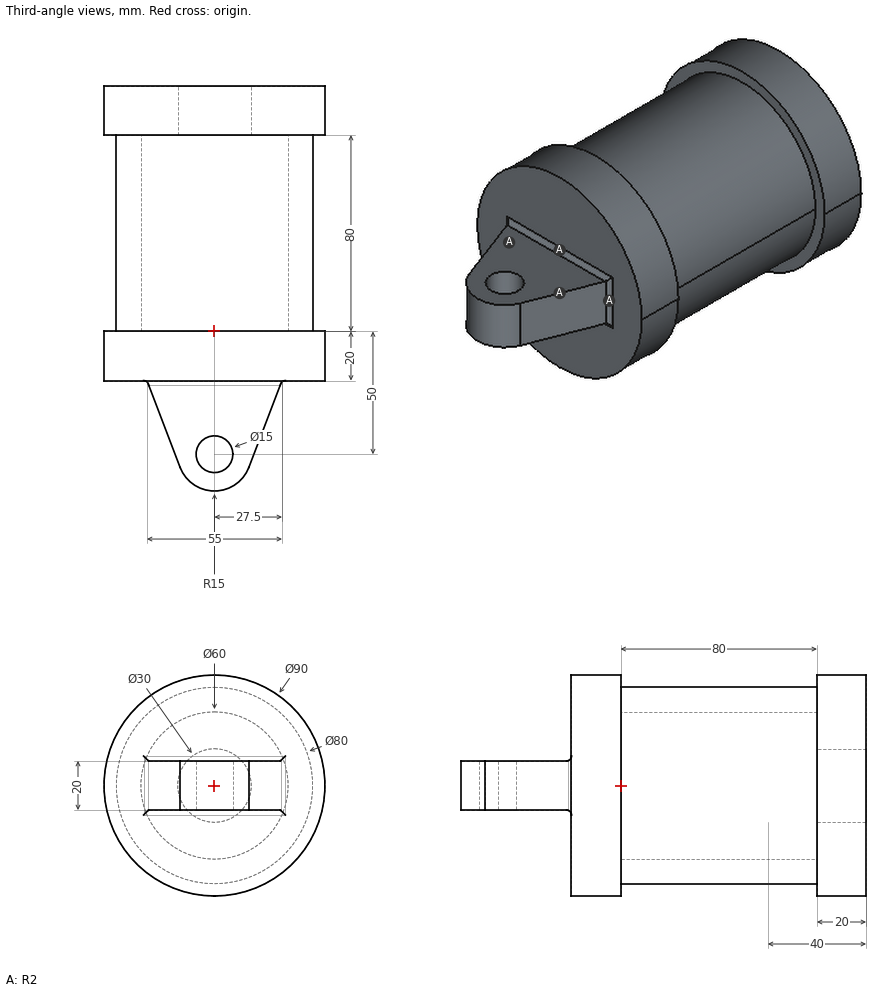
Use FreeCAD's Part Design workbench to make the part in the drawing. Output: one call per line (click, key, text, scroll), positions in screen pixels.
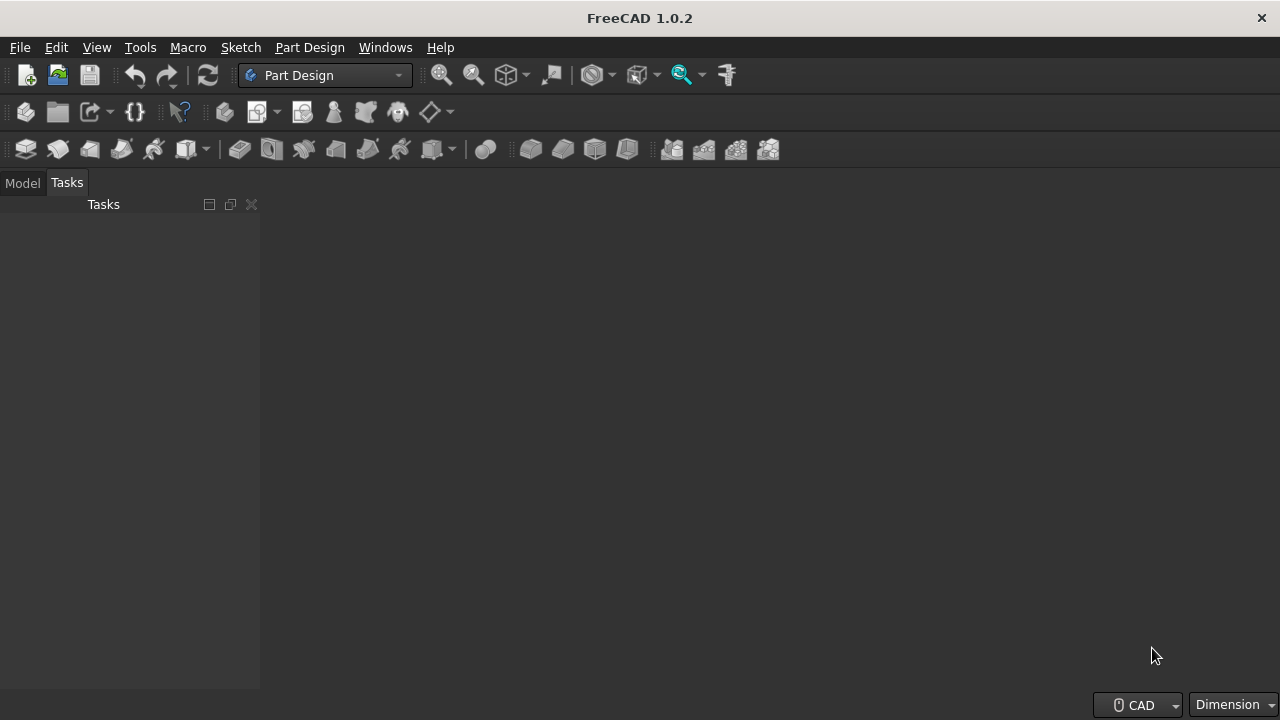
click(26, 76)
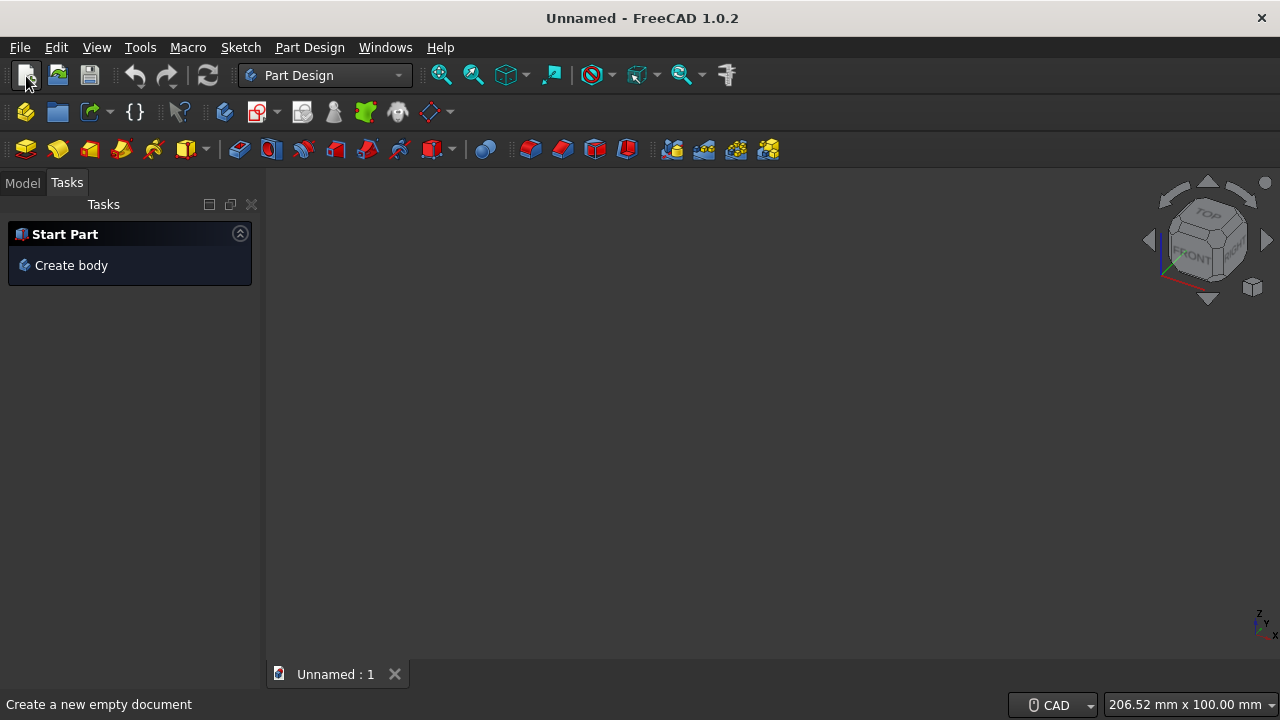
click(258, 112)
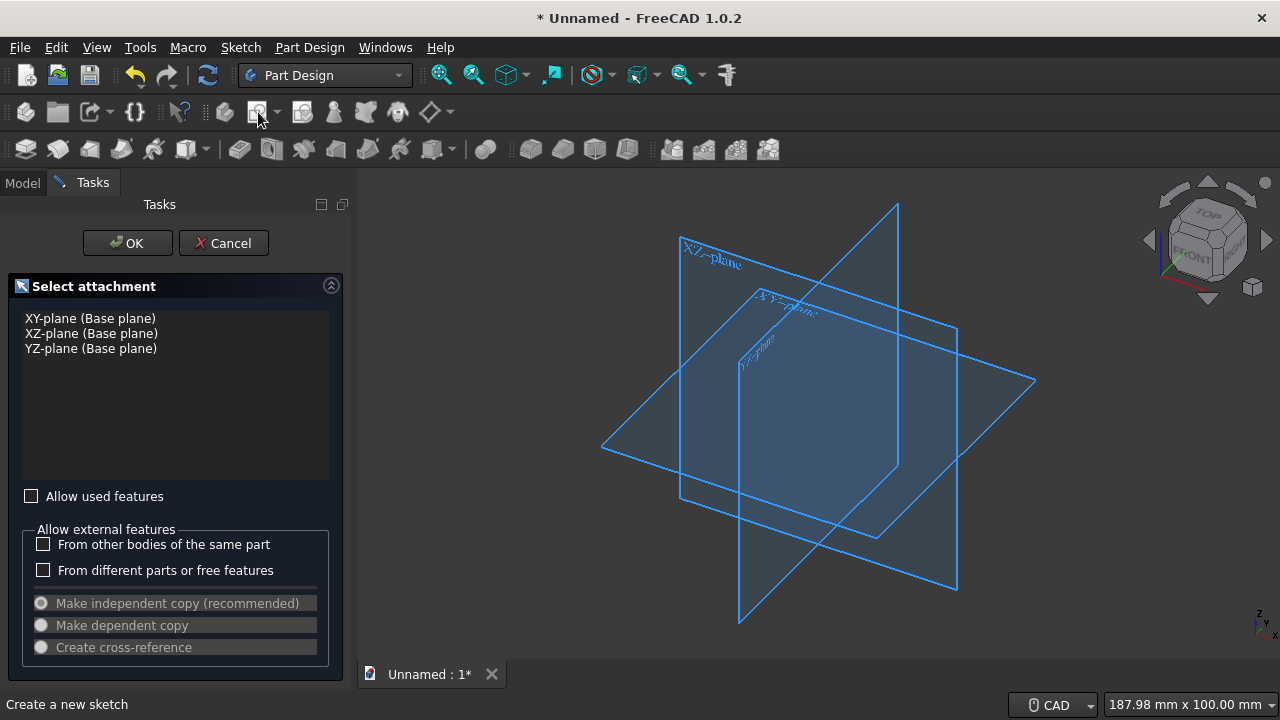
click(82, 334)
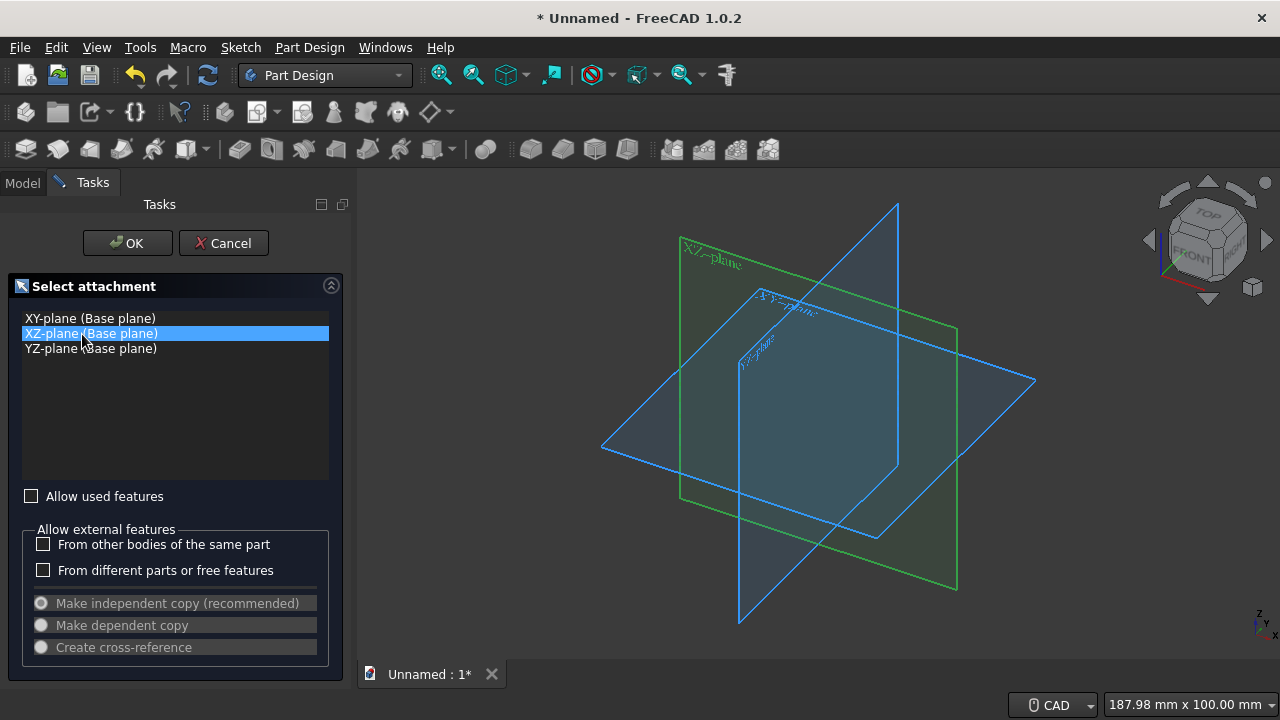
click(128, 243)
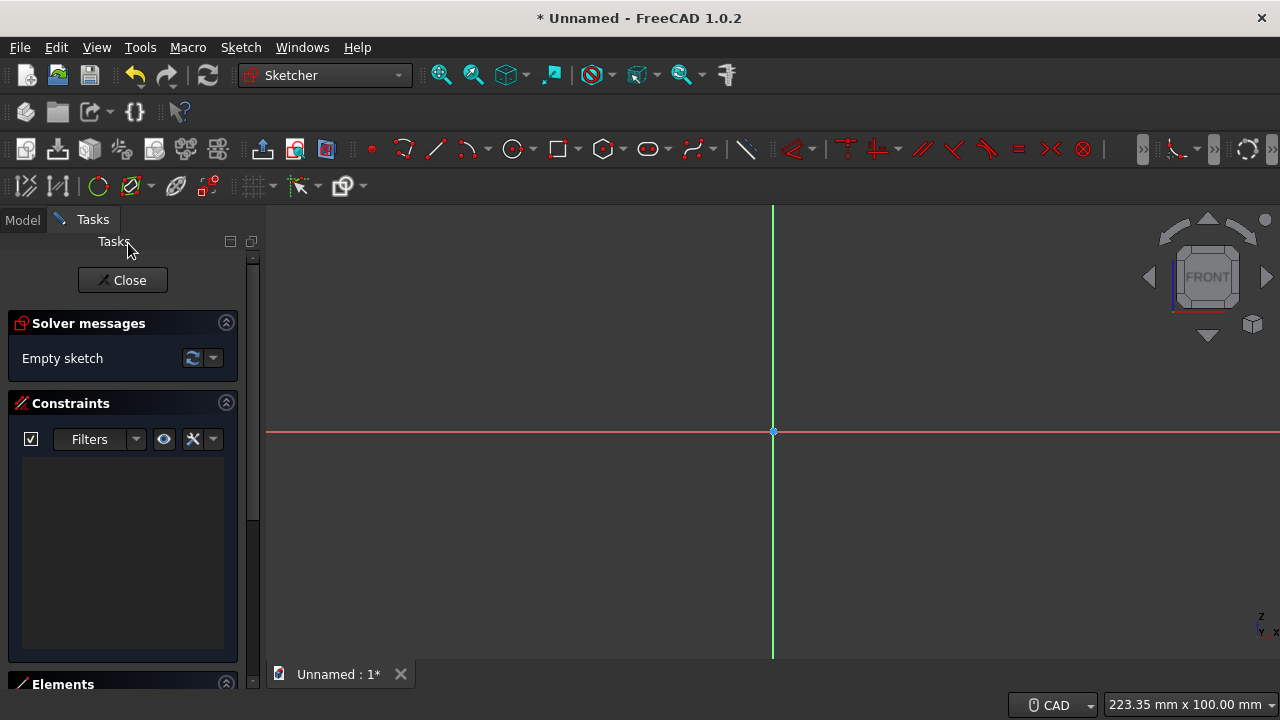
scroll(395, 432, down, 1)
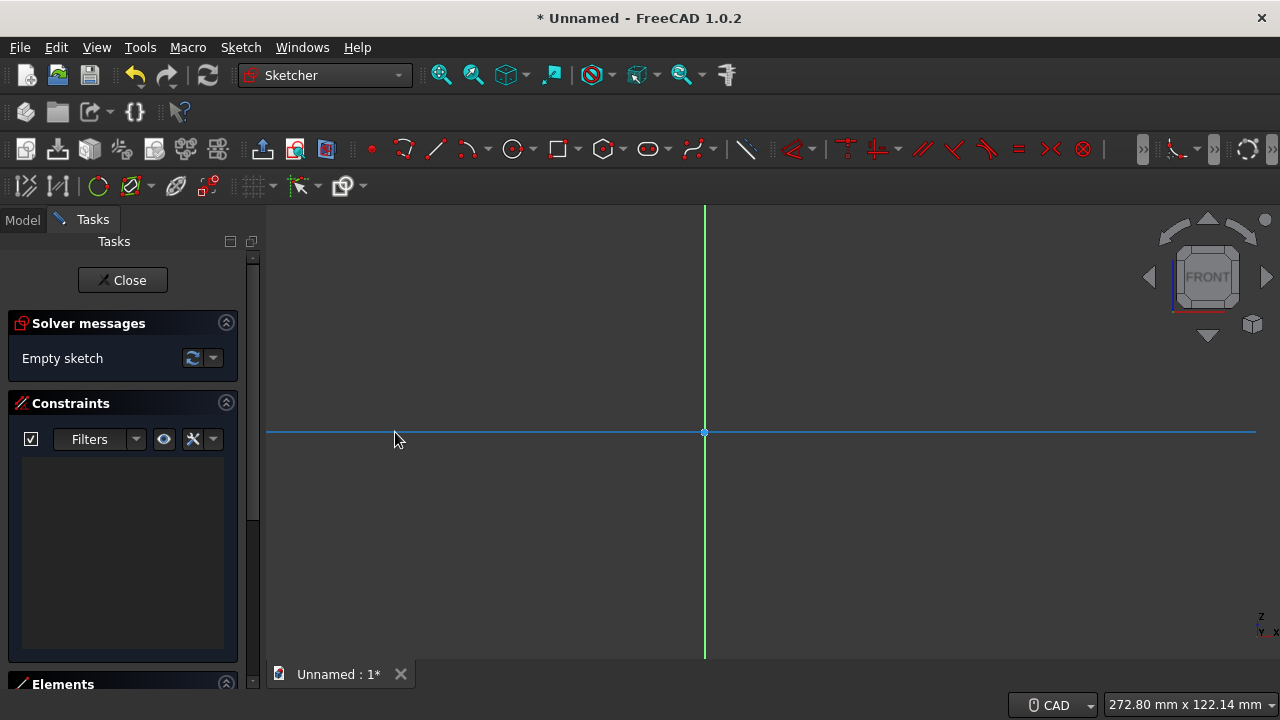
key(g)
key(c)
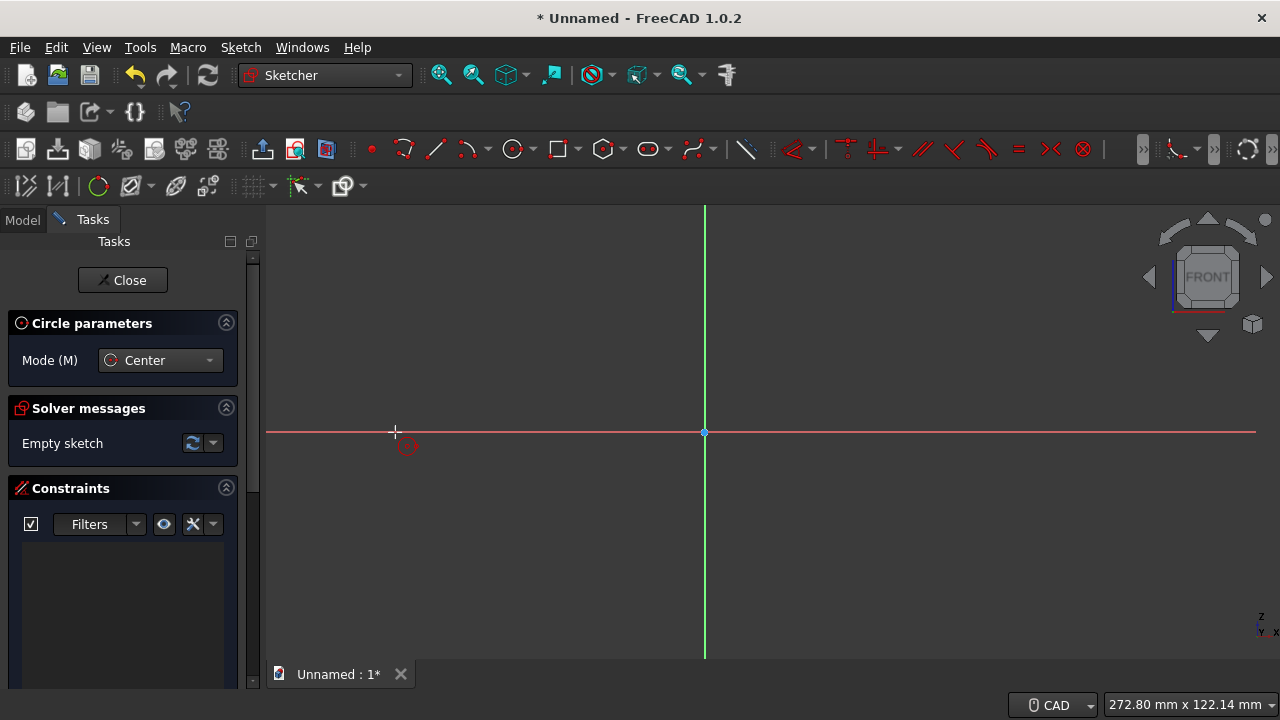
click(705, 432)
move(810, 327)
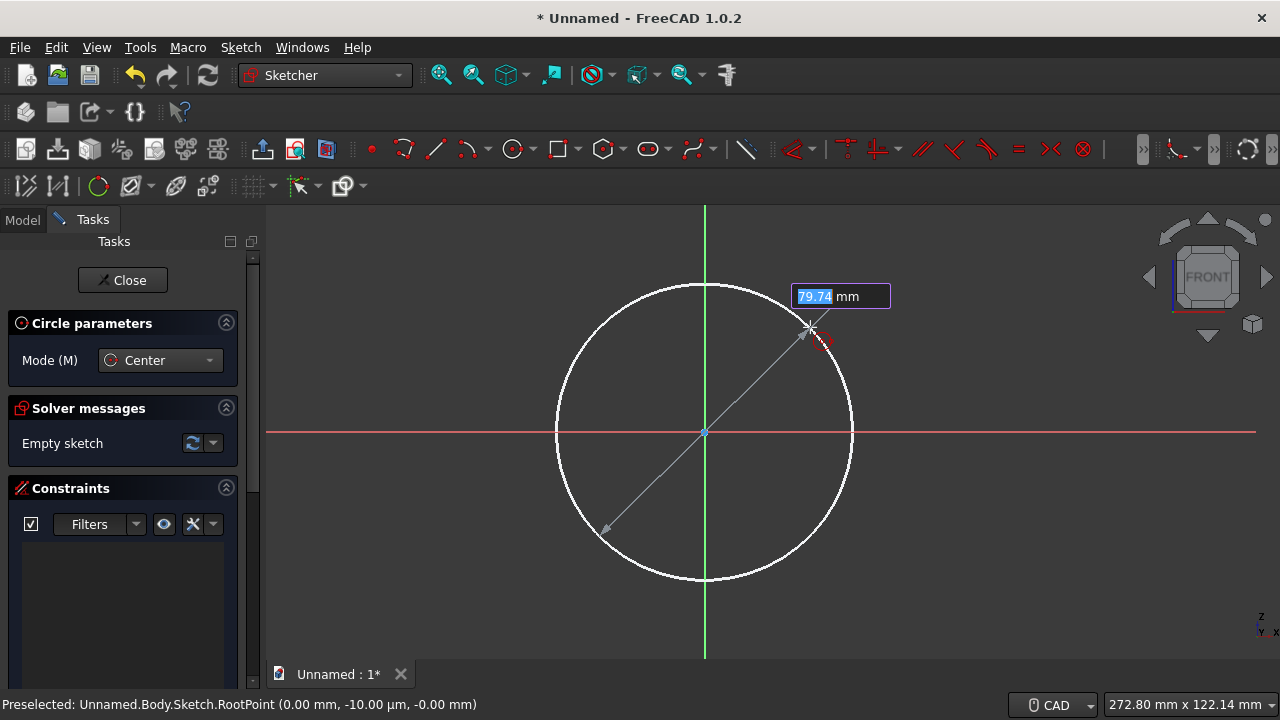
text(80)
key(Return)
key(Escape)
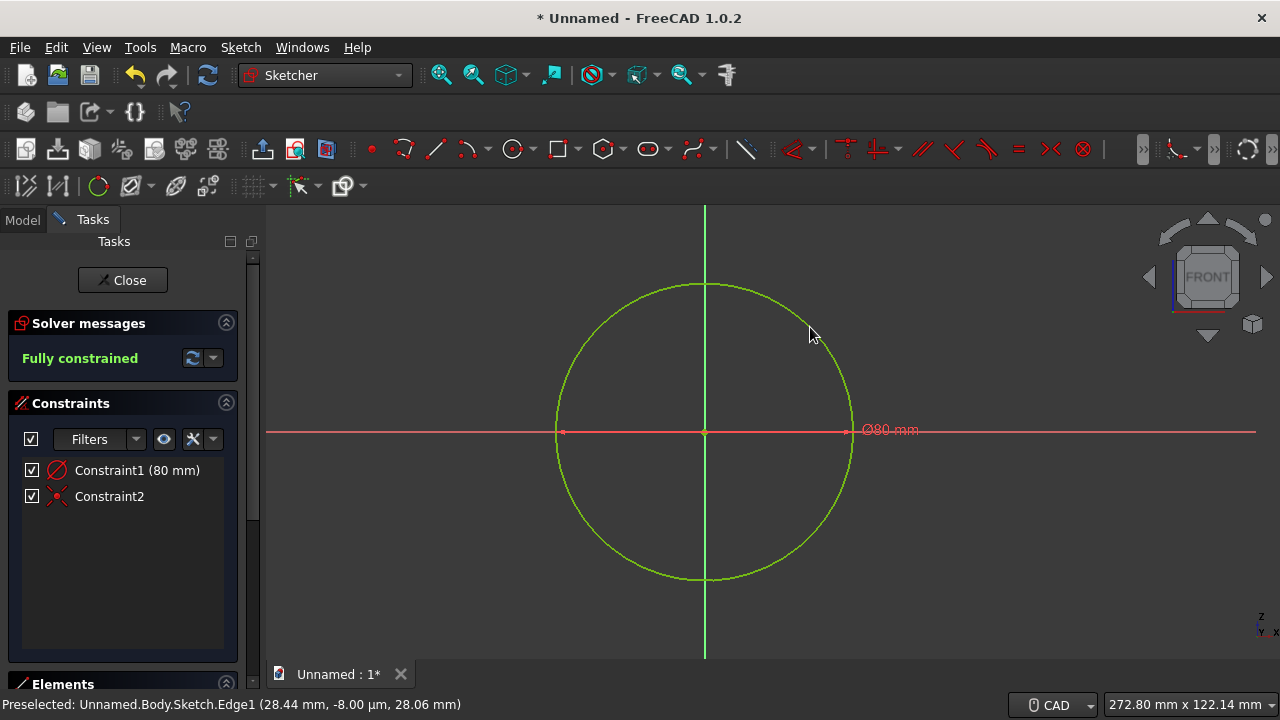
click(123, 280)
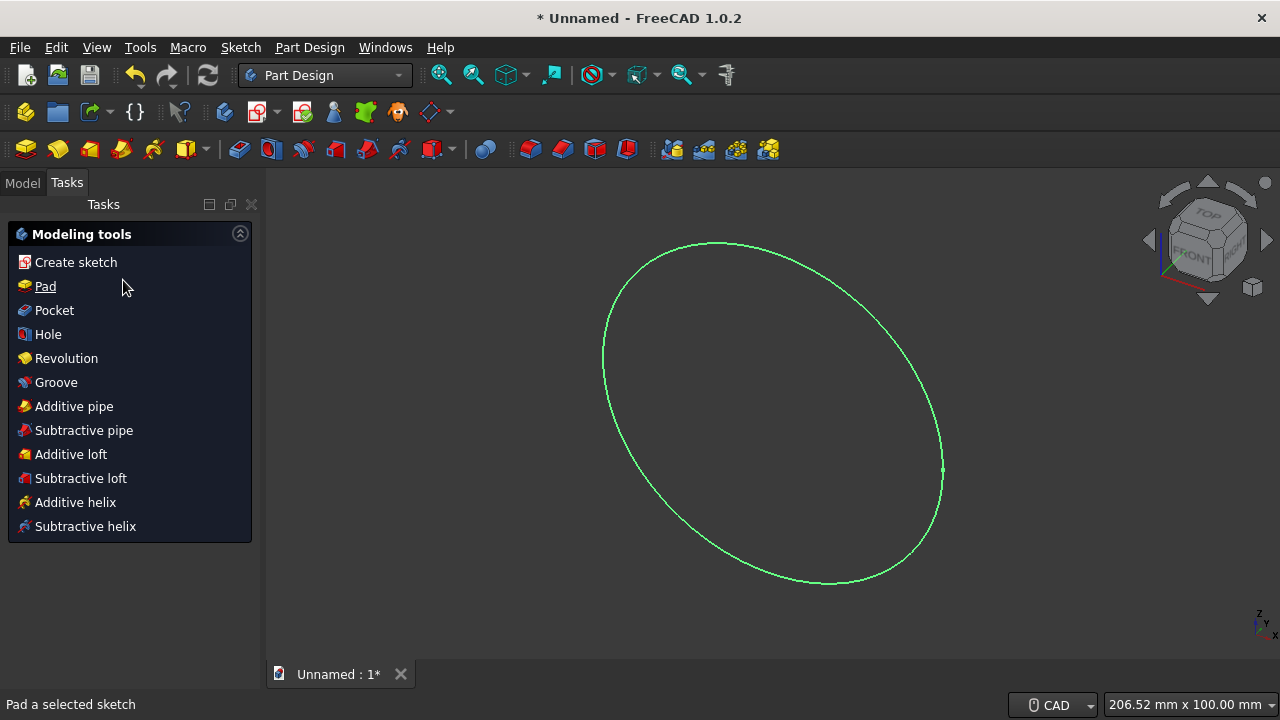
click(26, 150)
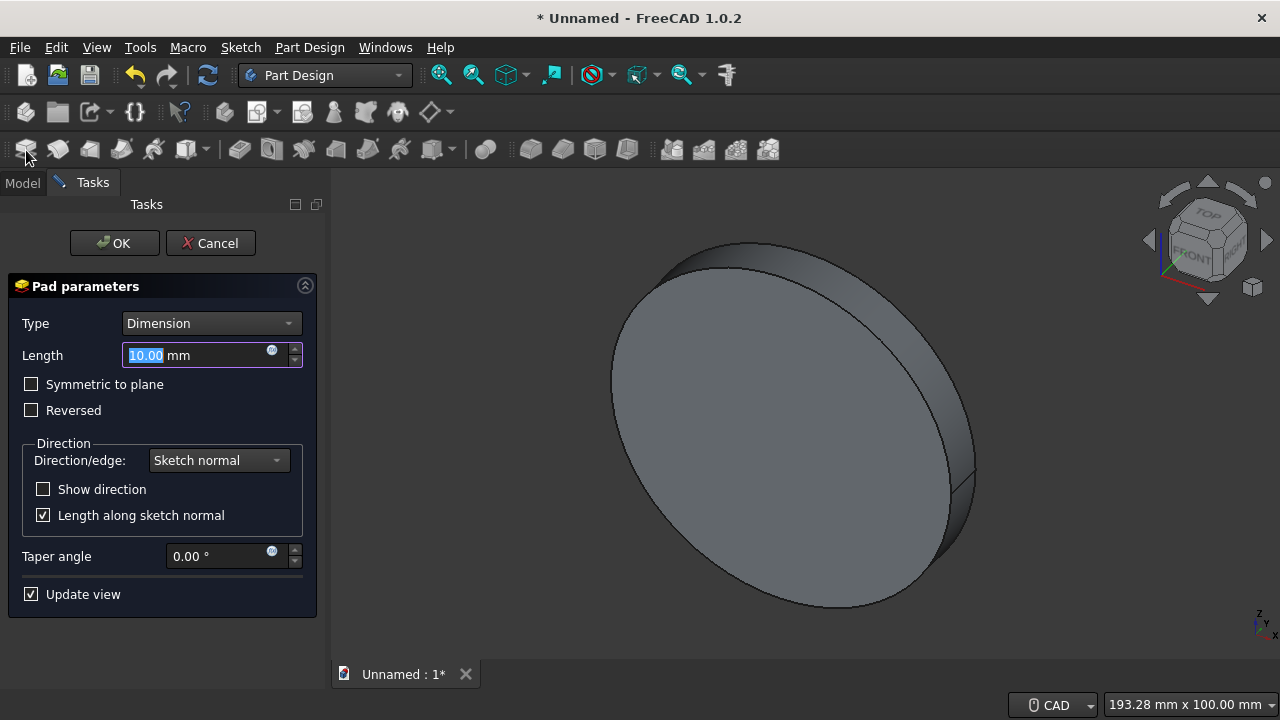
text(80)
key(Tab)